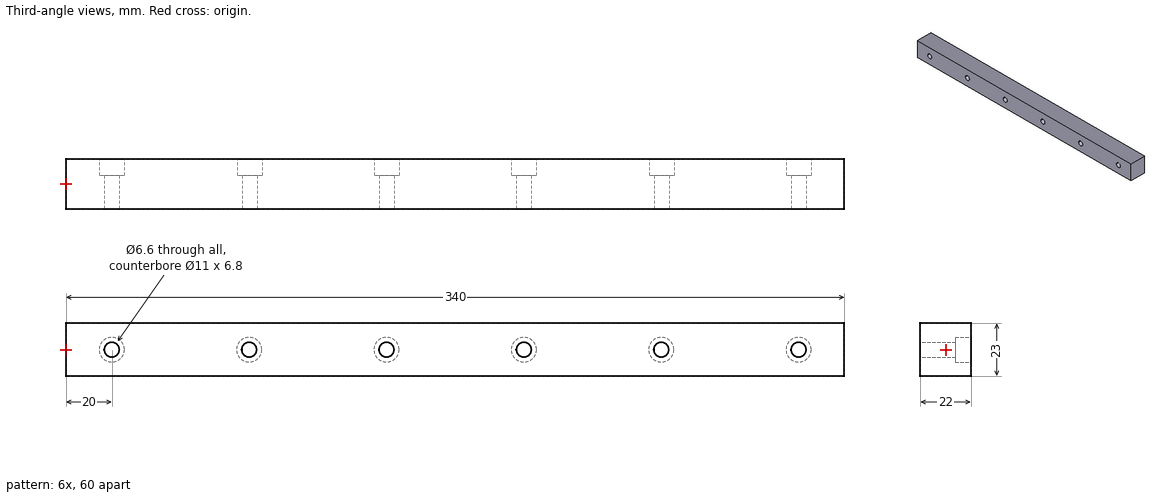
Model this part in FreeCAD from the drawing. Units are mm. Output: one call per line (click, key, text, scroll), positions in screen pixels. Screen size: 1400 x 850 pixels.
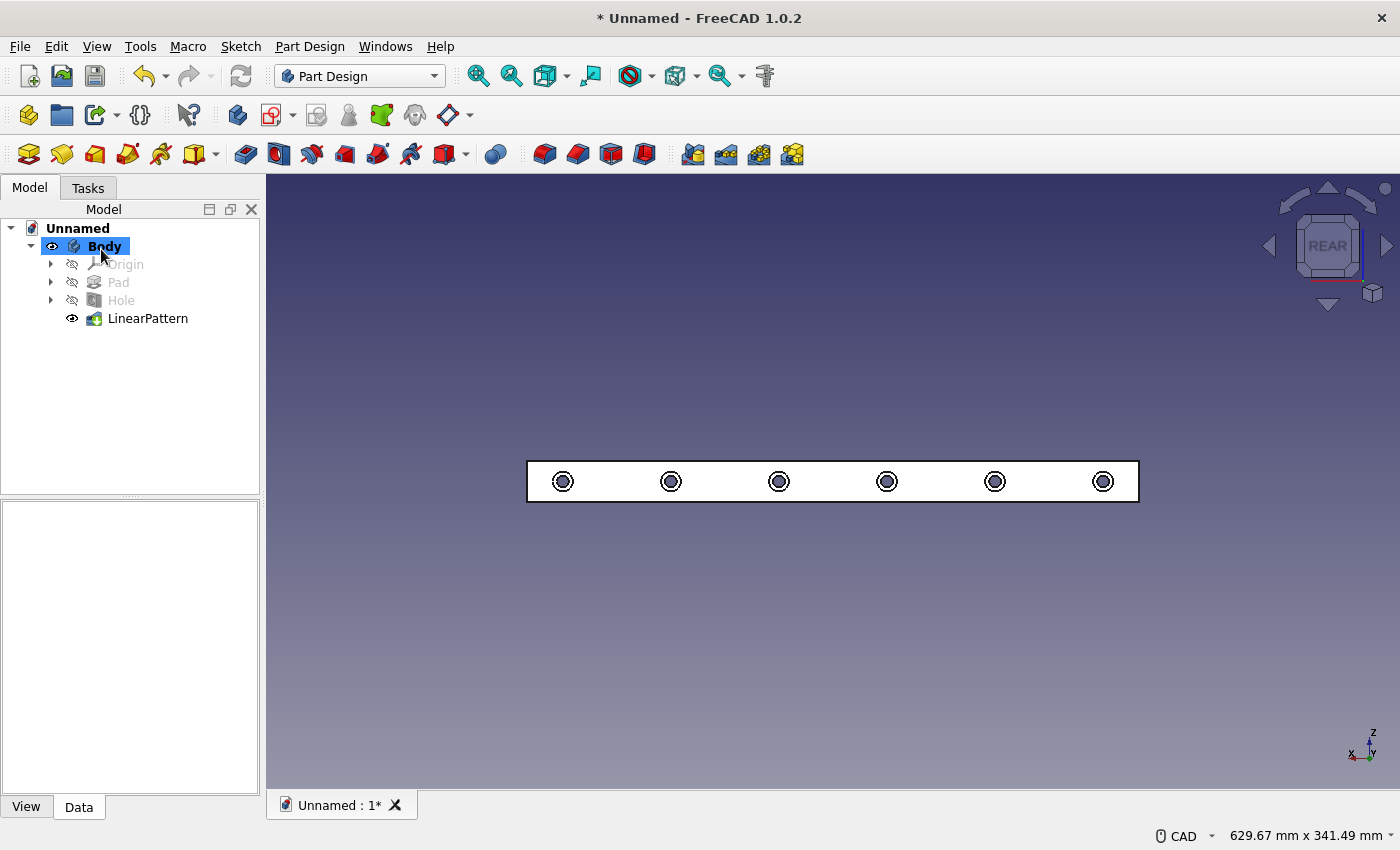
key(0)